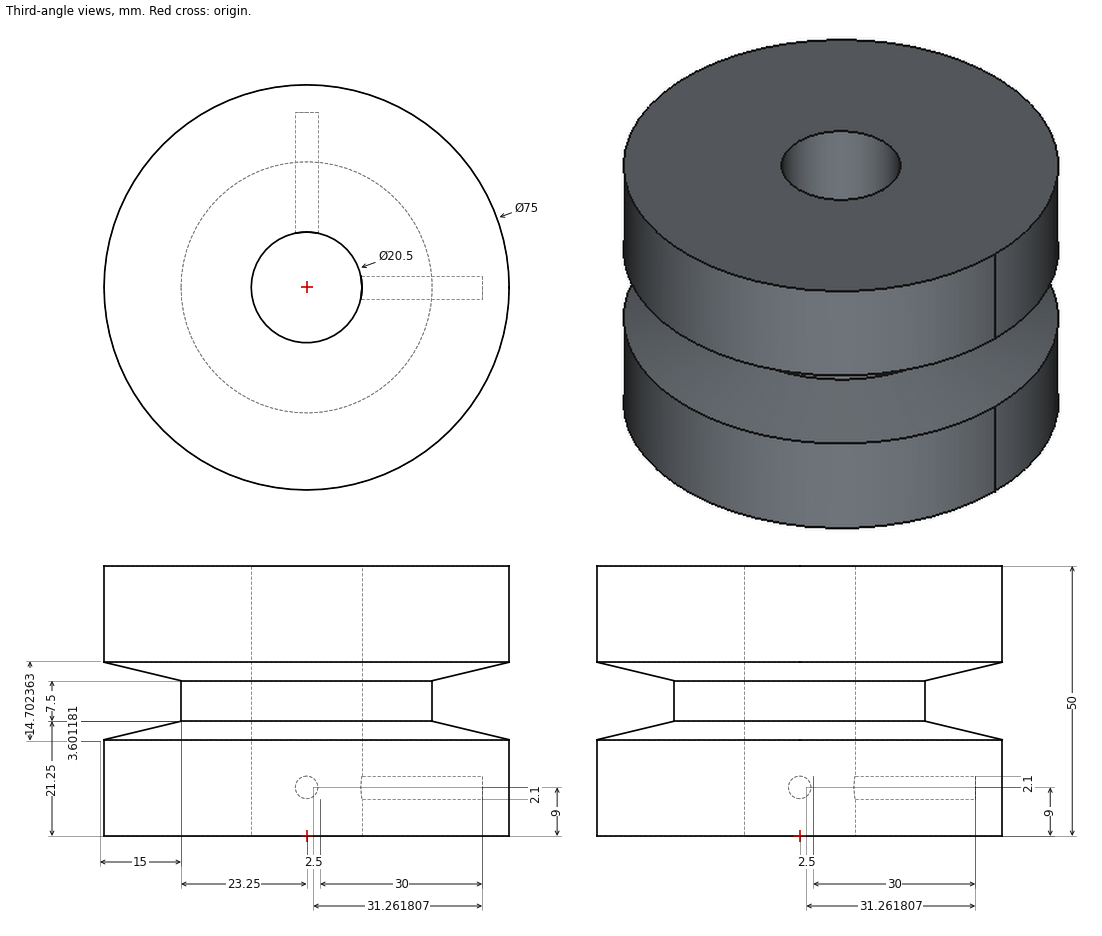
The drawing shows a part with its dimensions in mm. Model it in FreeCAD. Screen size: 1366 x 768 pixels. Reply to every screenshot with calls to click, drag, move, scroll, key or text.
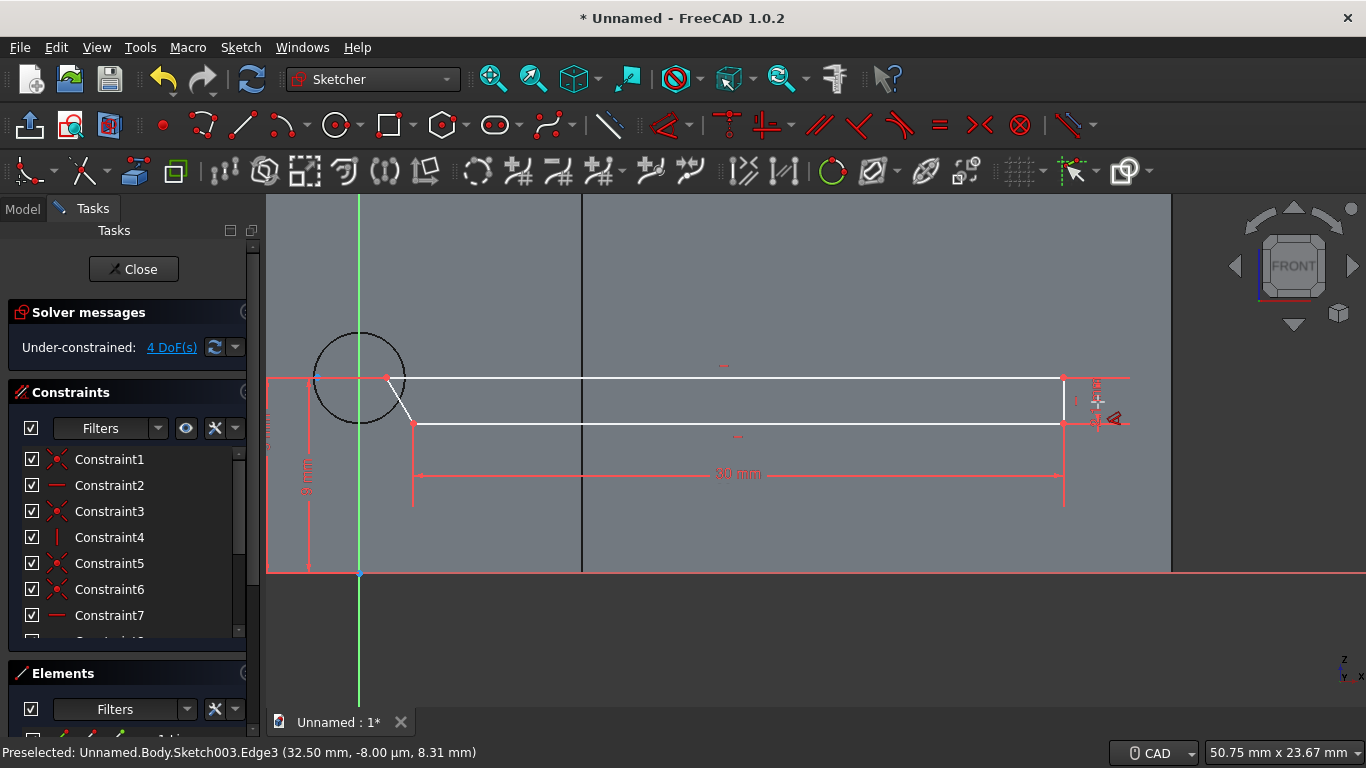
click(413, 423)
click(386, 607)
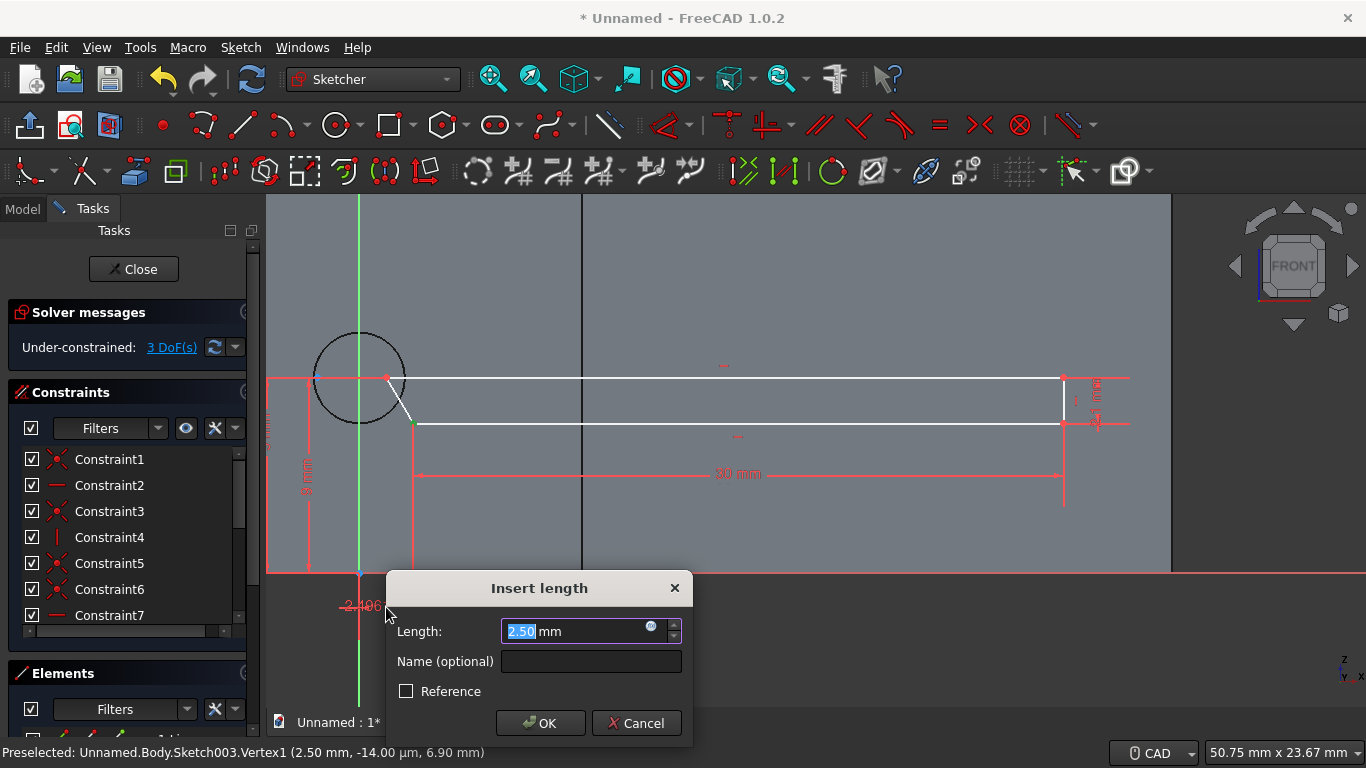
text(2.5)
key(Return)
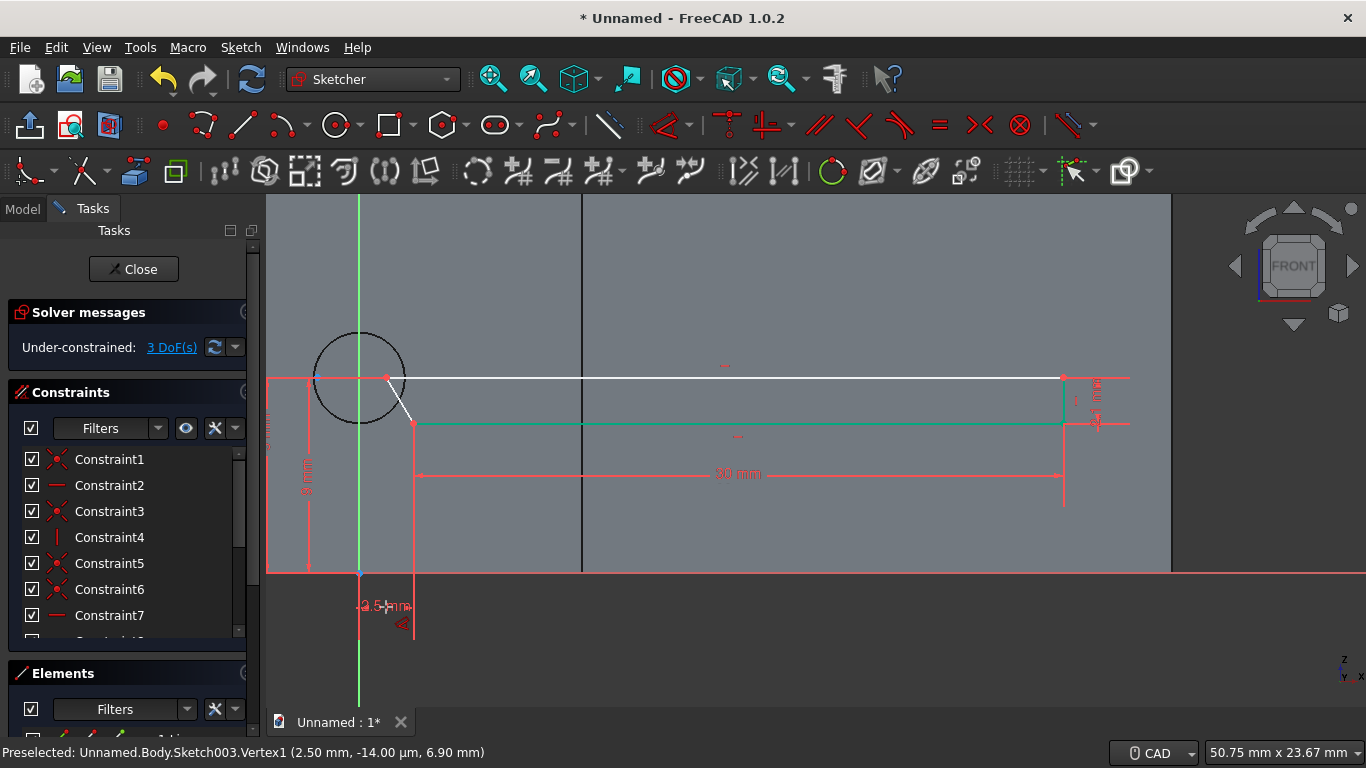
click(590, 378)
click(725, 344)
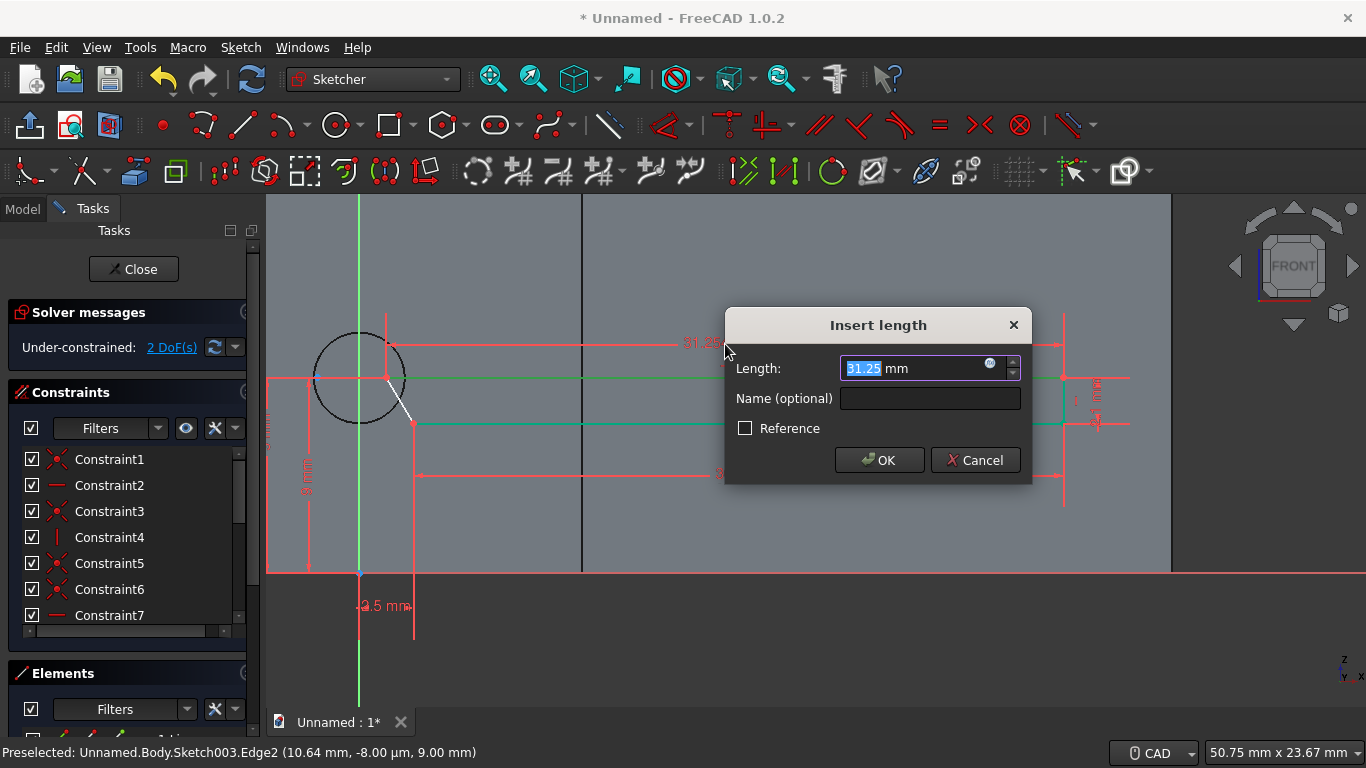
text(31.261807)
key(Return)
key(Escape)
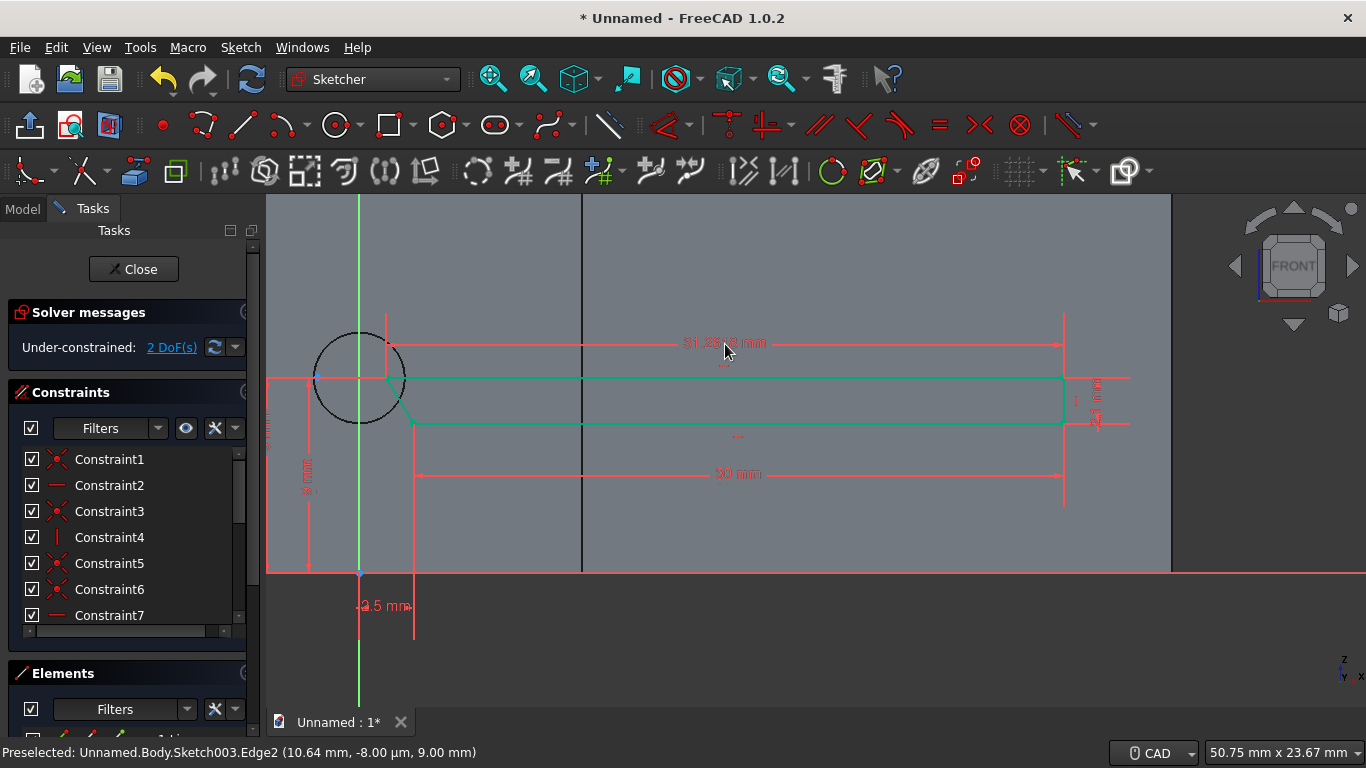
click(134, 269)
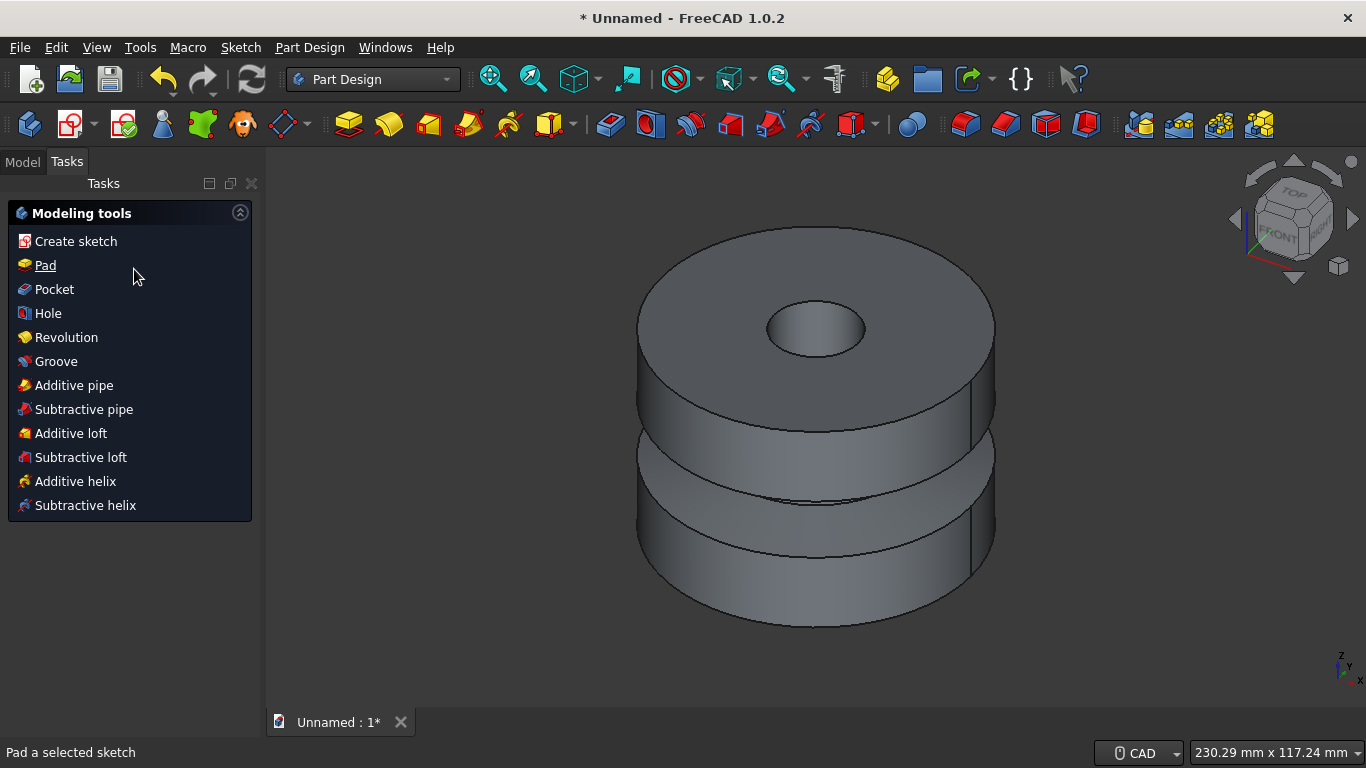
click(692, 124)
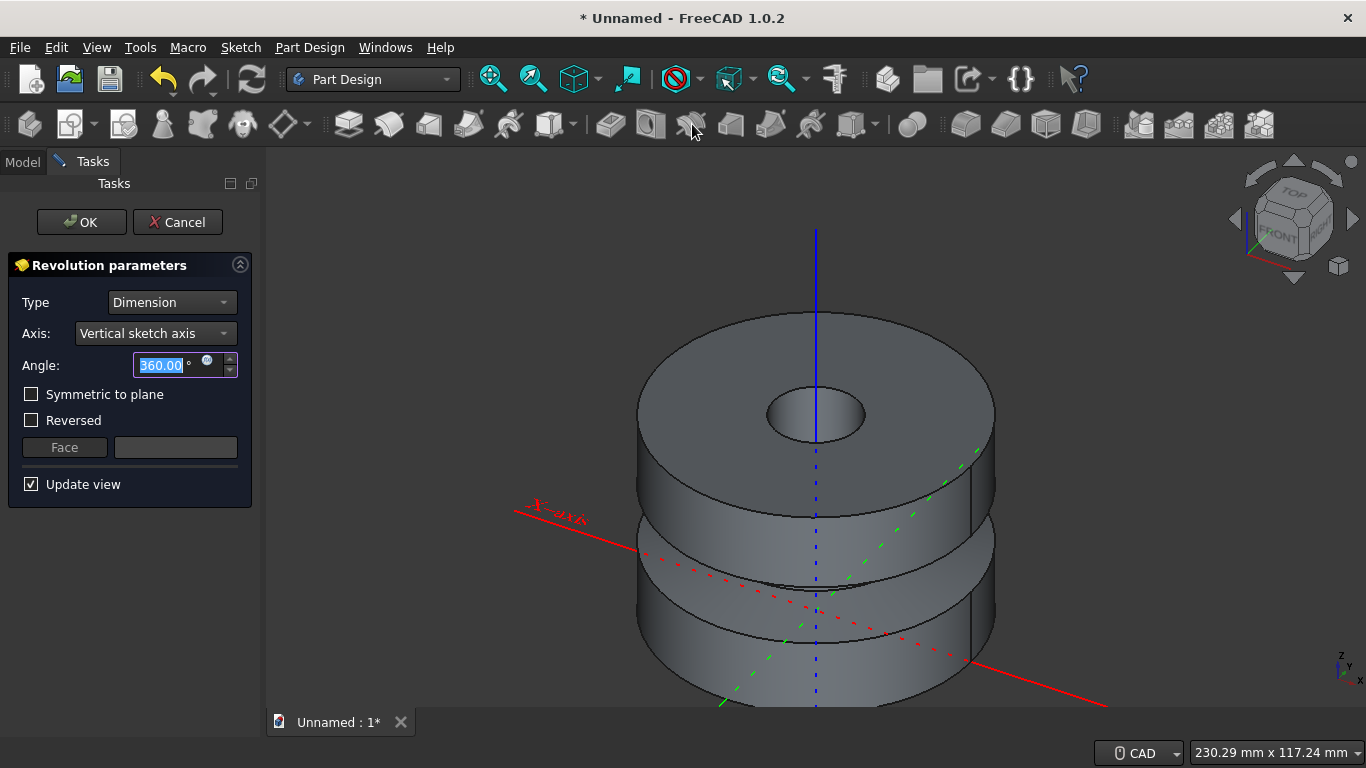
click(156, 334)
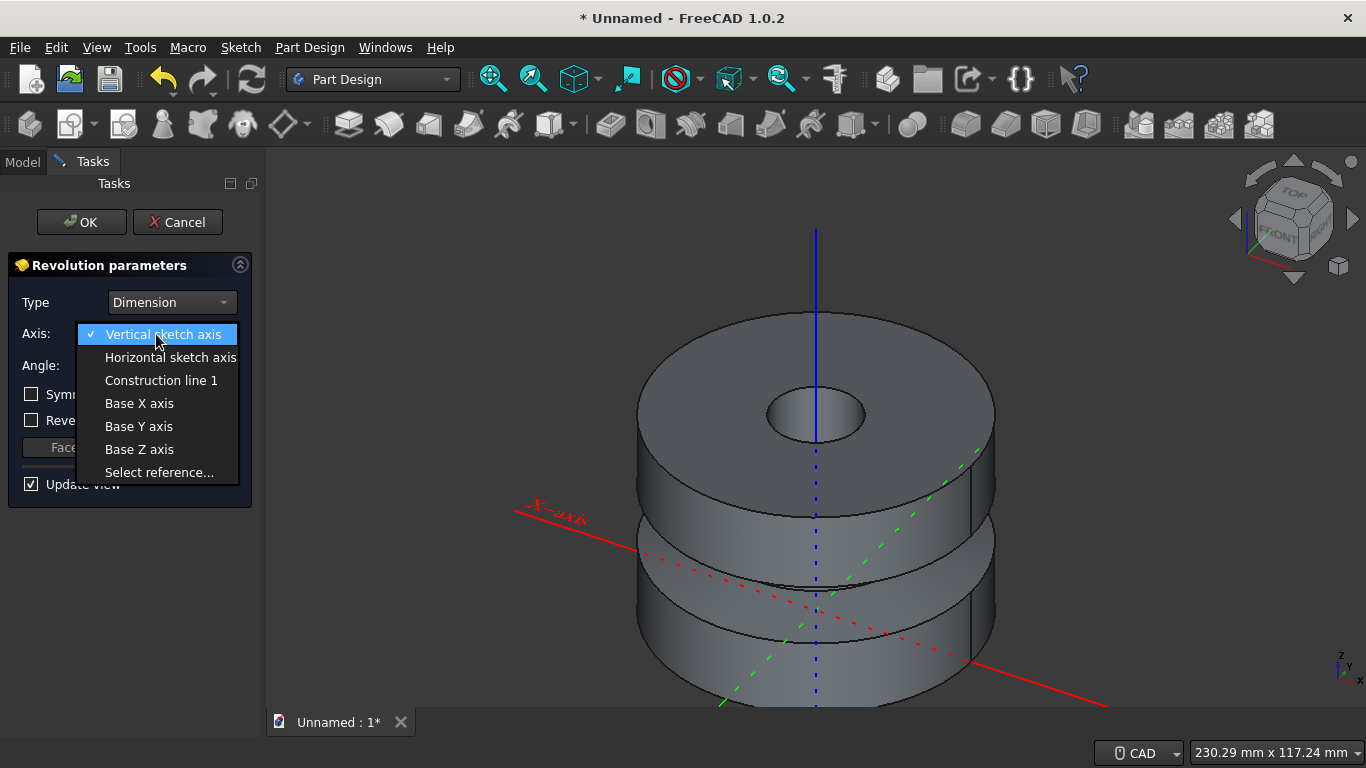
click(156, 380)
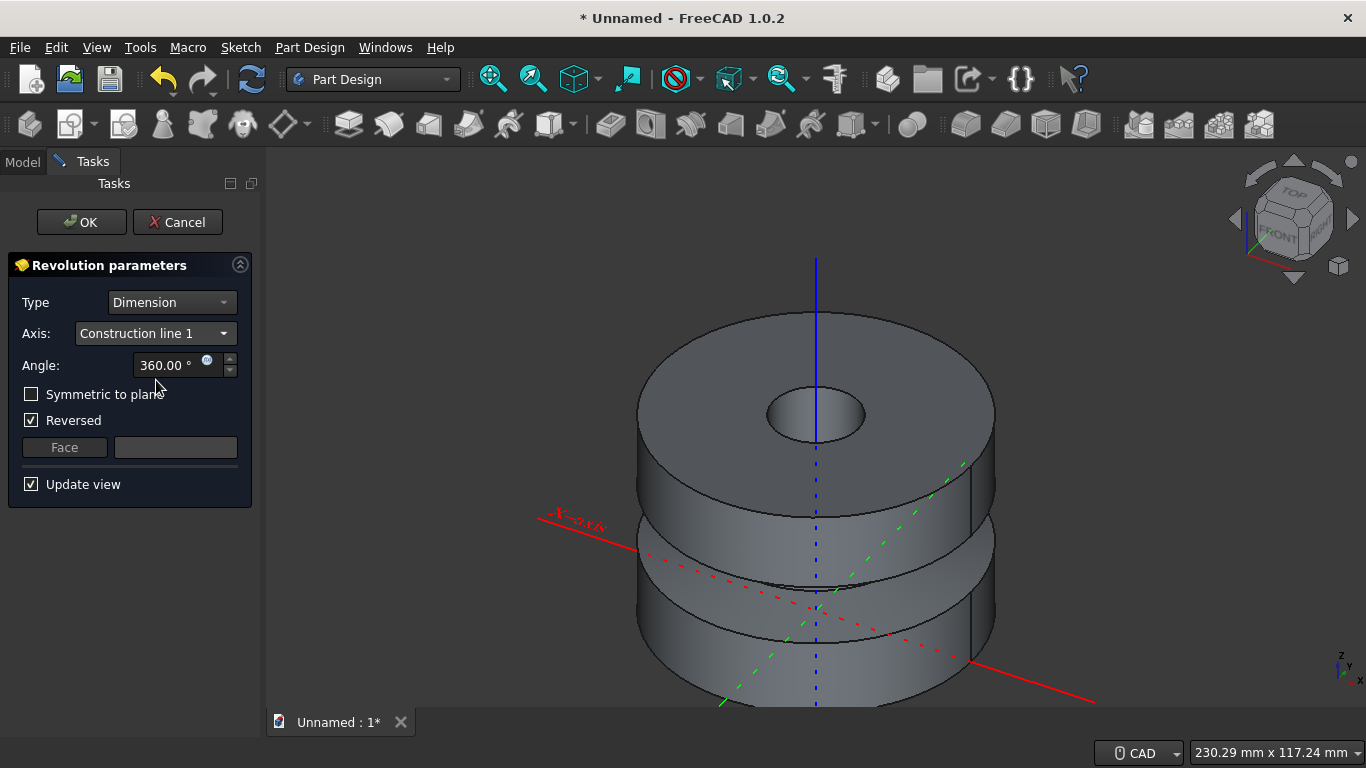
click(82, 222)